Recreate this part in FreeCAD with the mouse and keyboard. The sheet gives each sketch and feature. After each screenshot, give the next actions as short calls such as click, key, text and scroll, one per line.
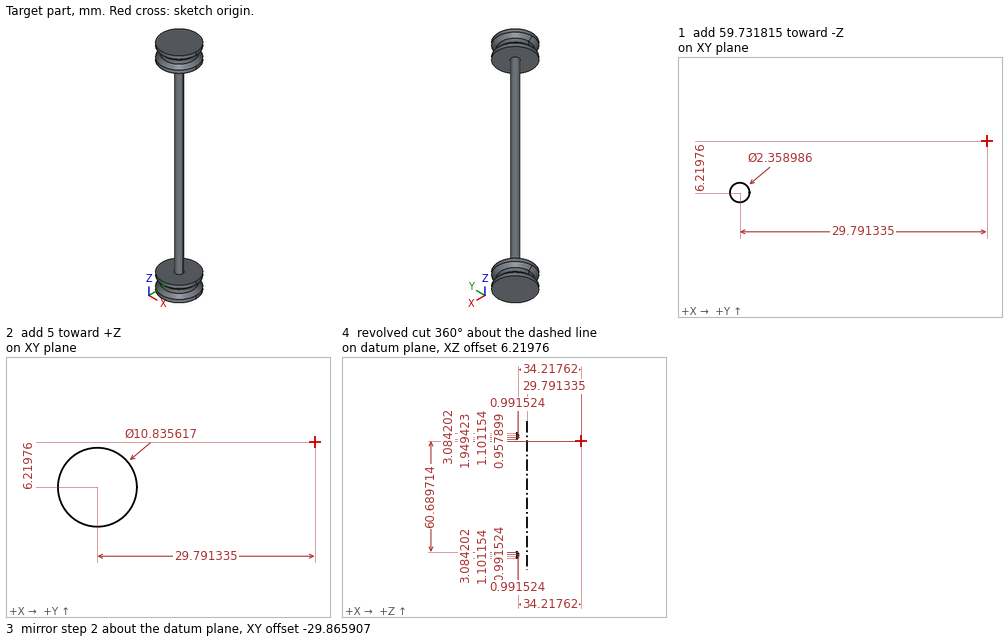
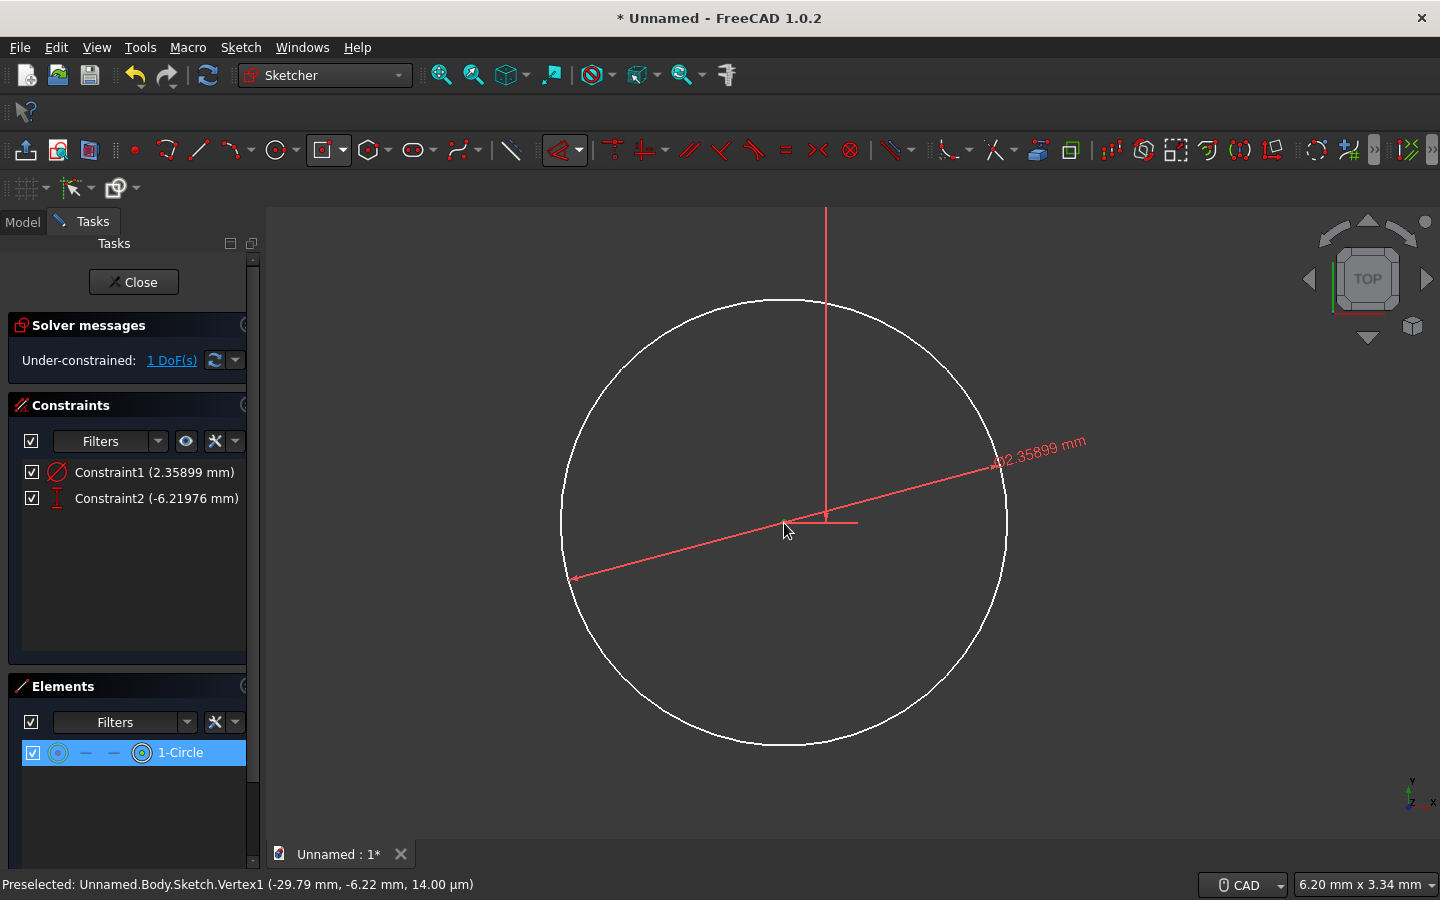
click(582, 150)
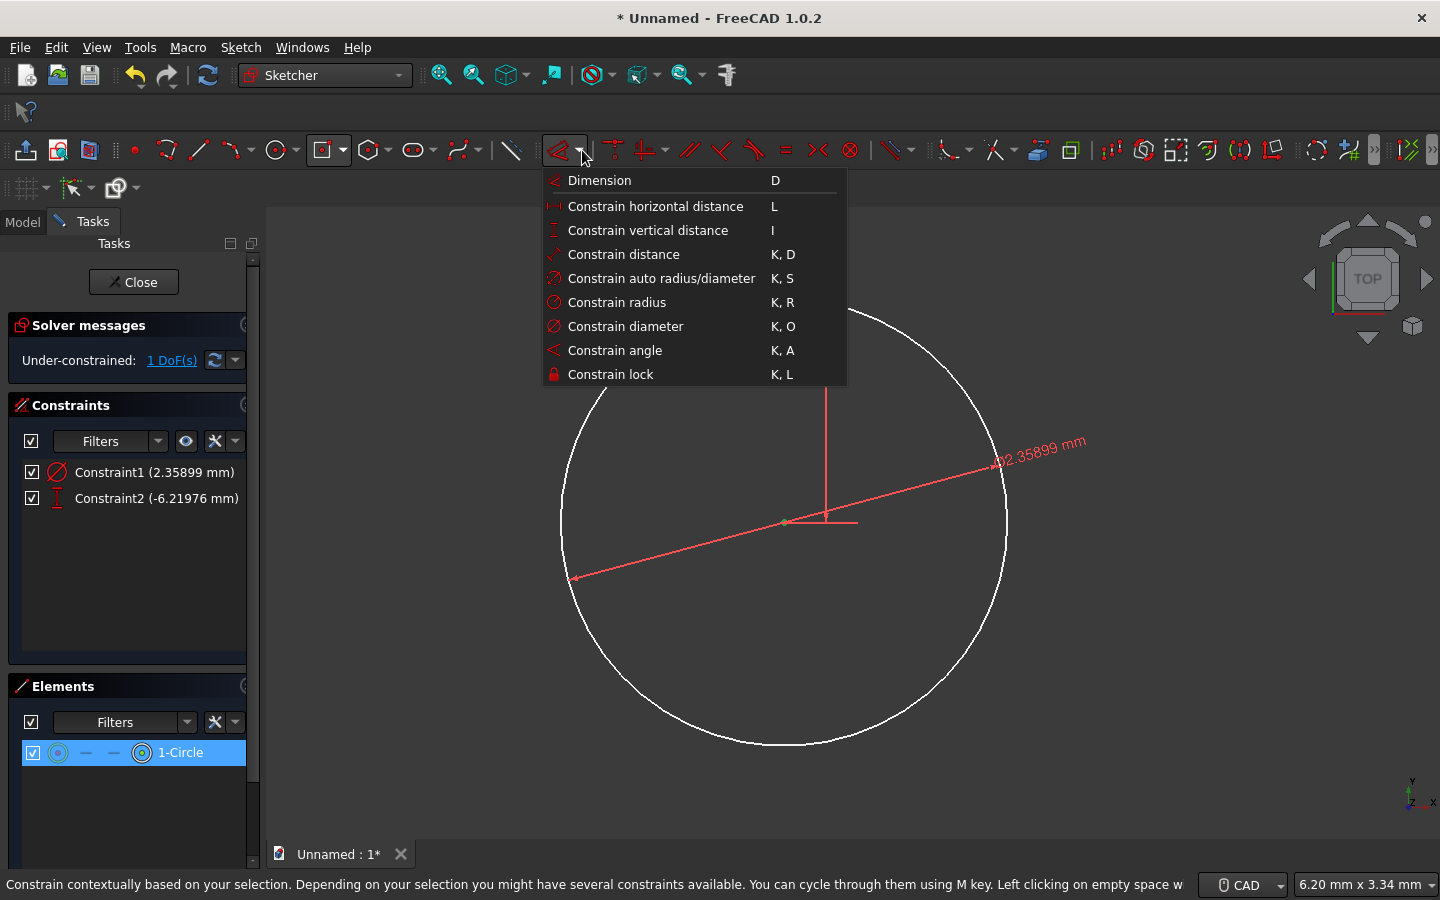
click(695, 206)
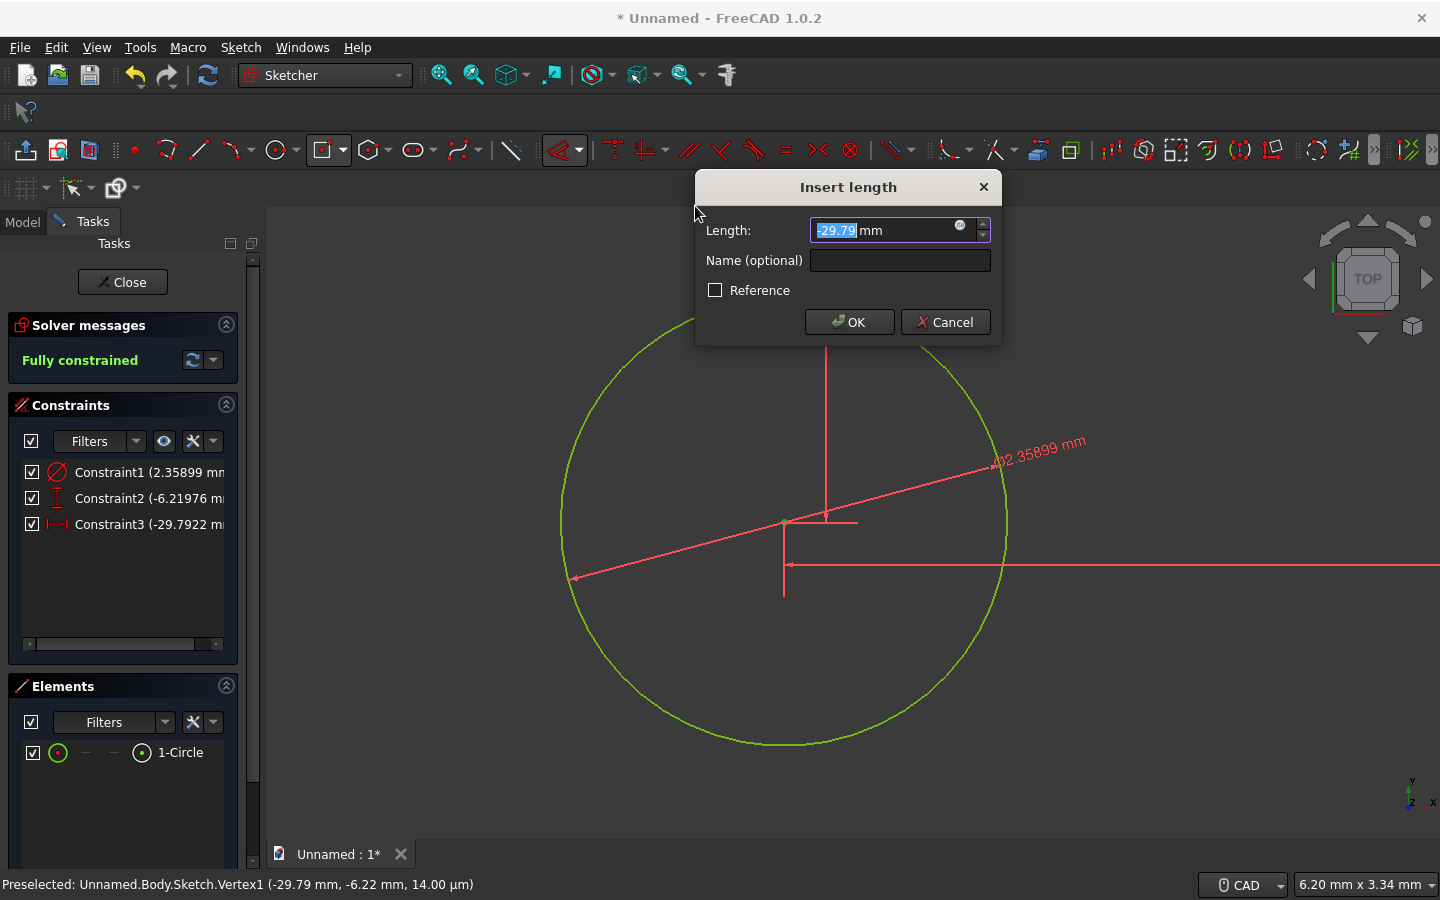
text(-29.791335)
key(Return)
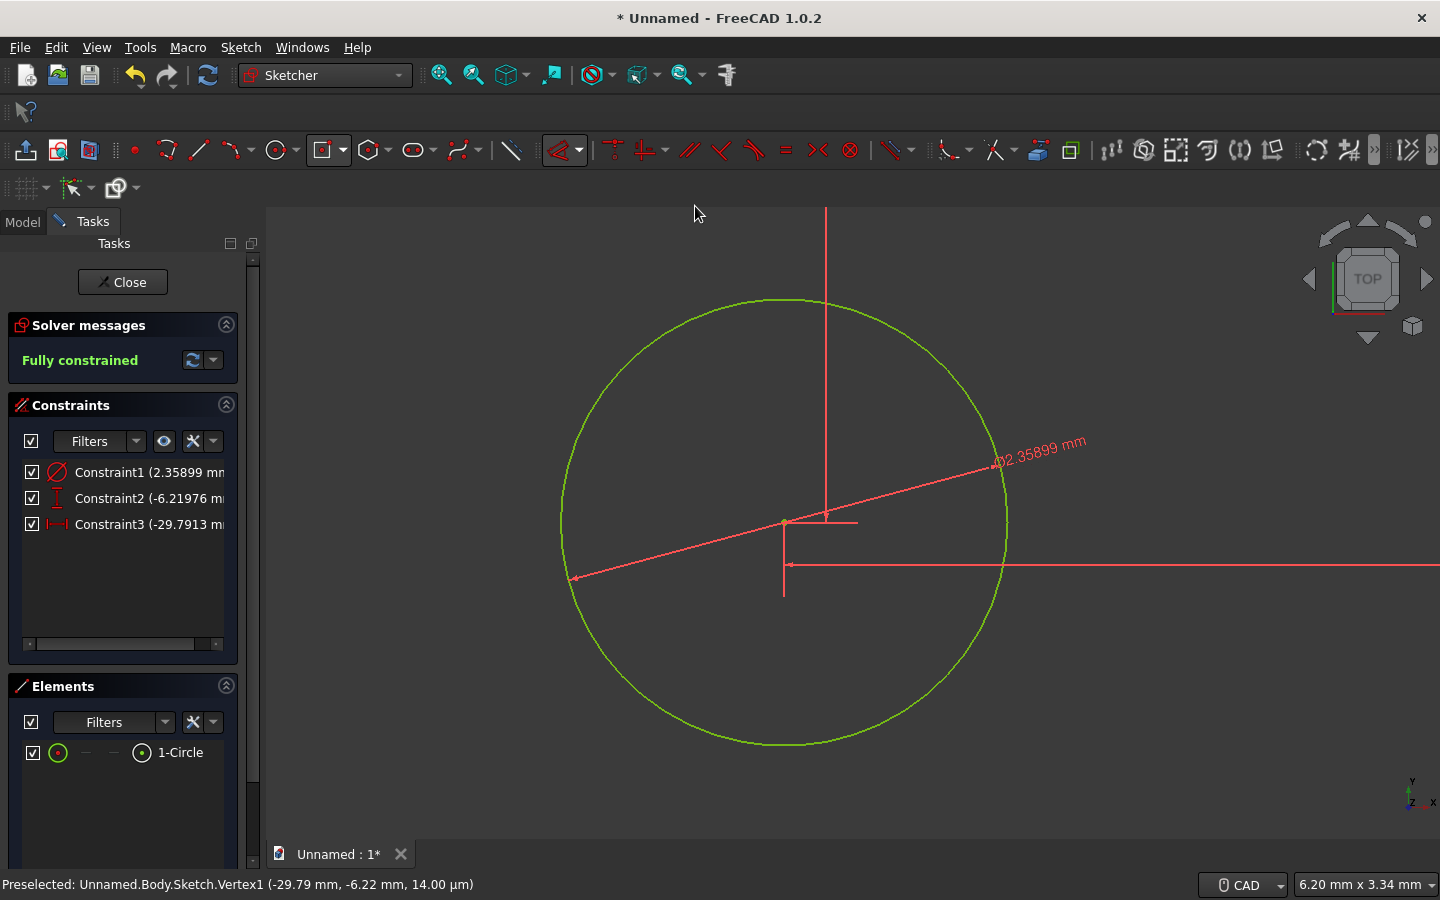
click(123, 282)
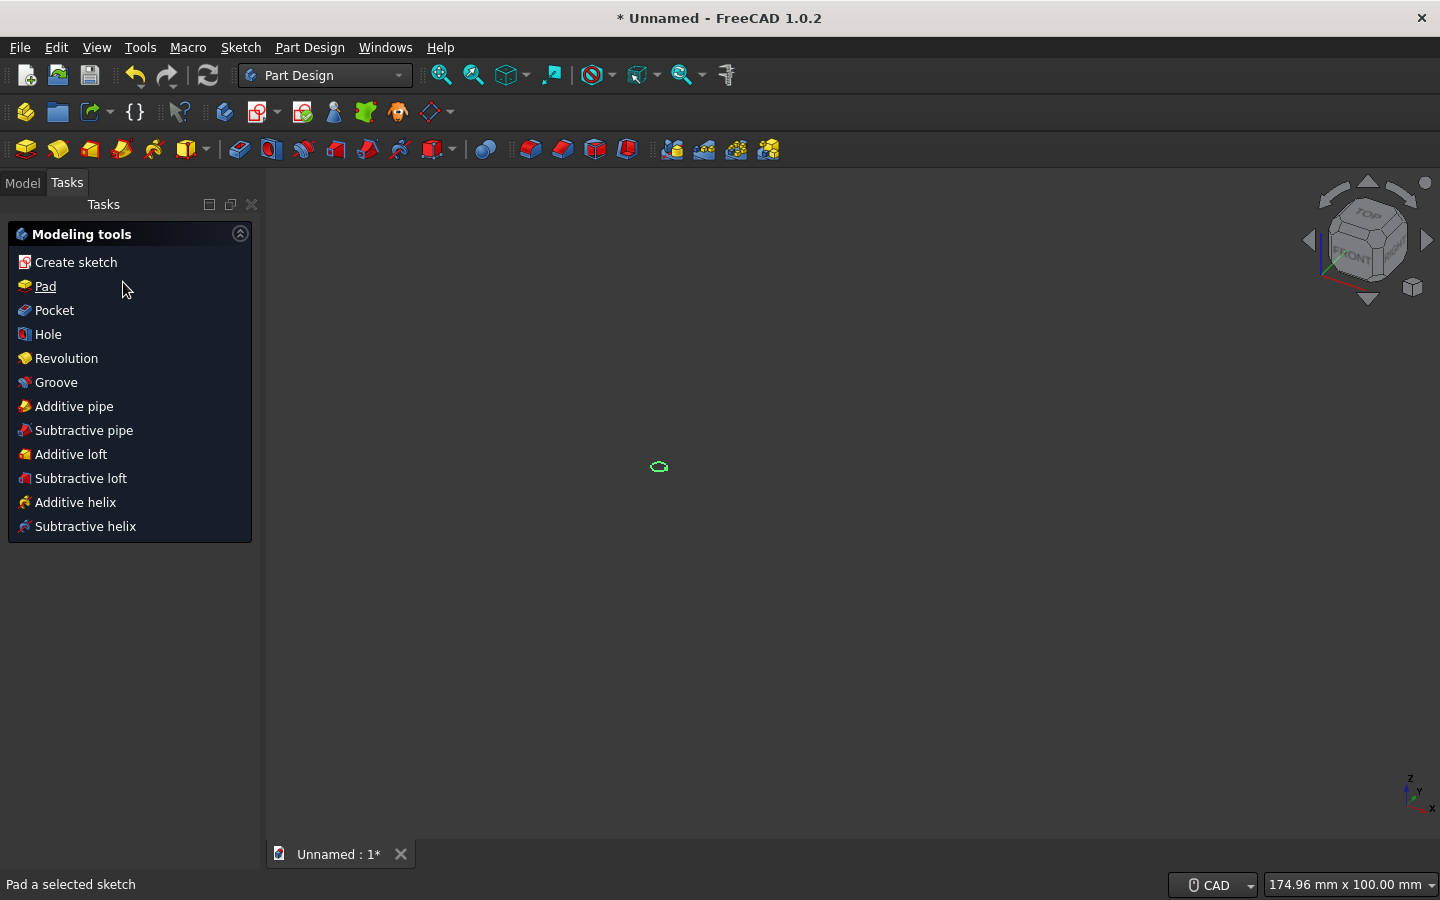
click(26, 150)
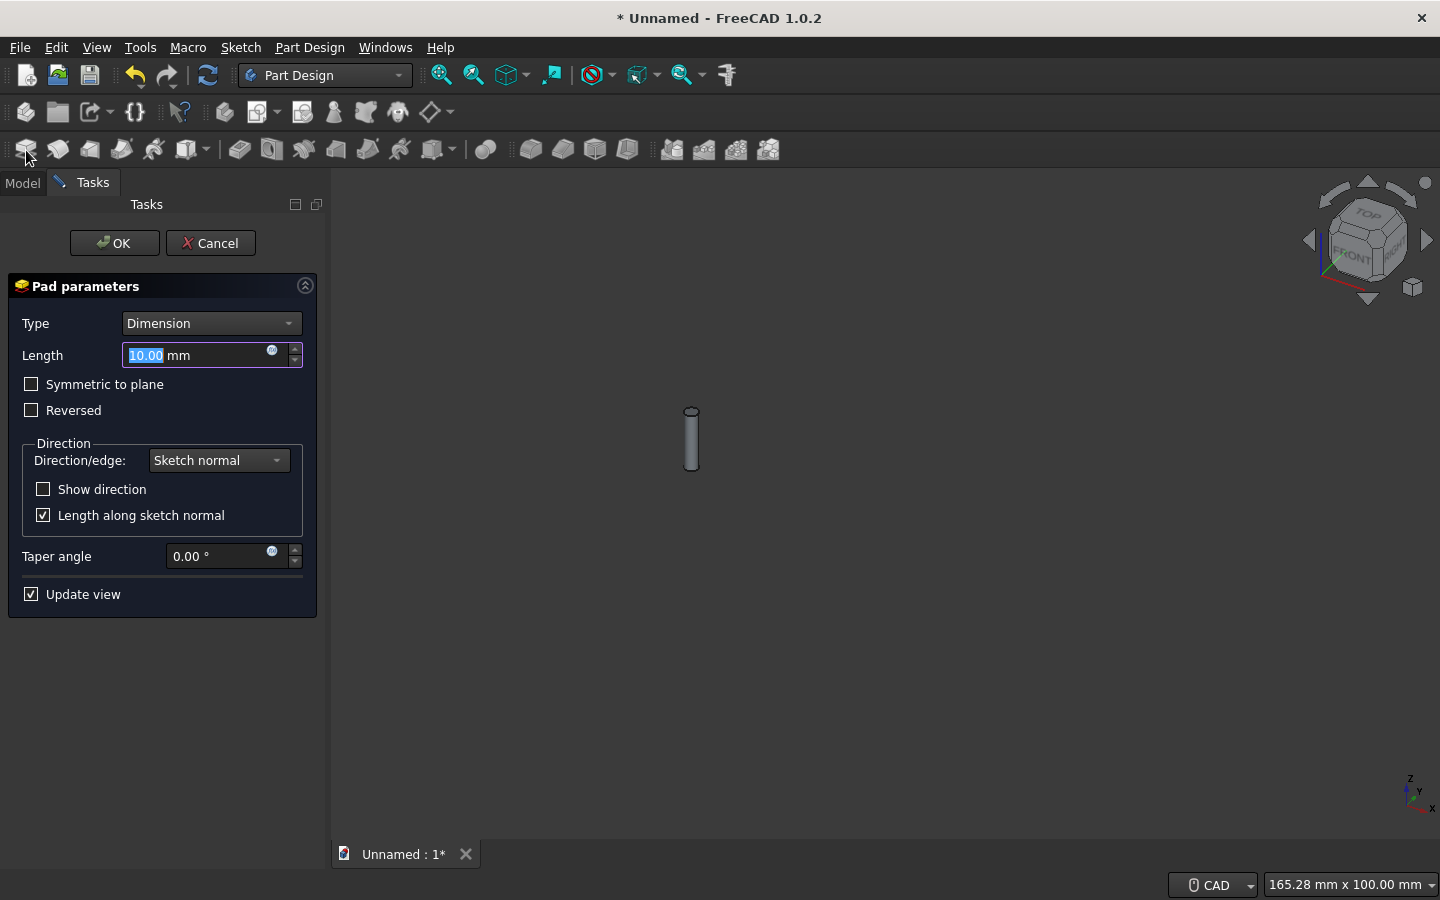
text(59.731815)
key(Tab)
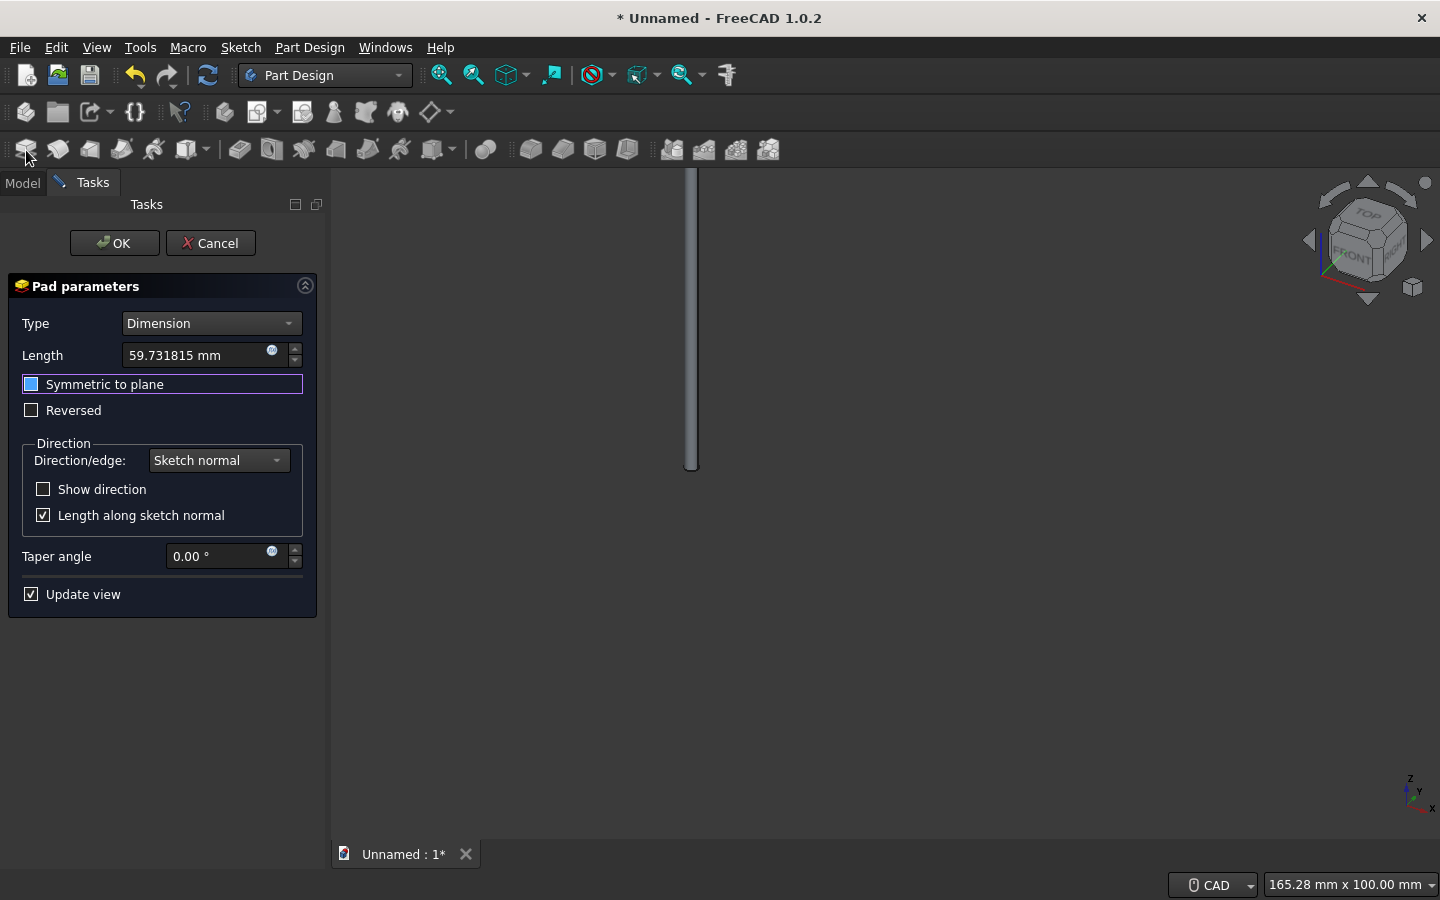
click(30, 410)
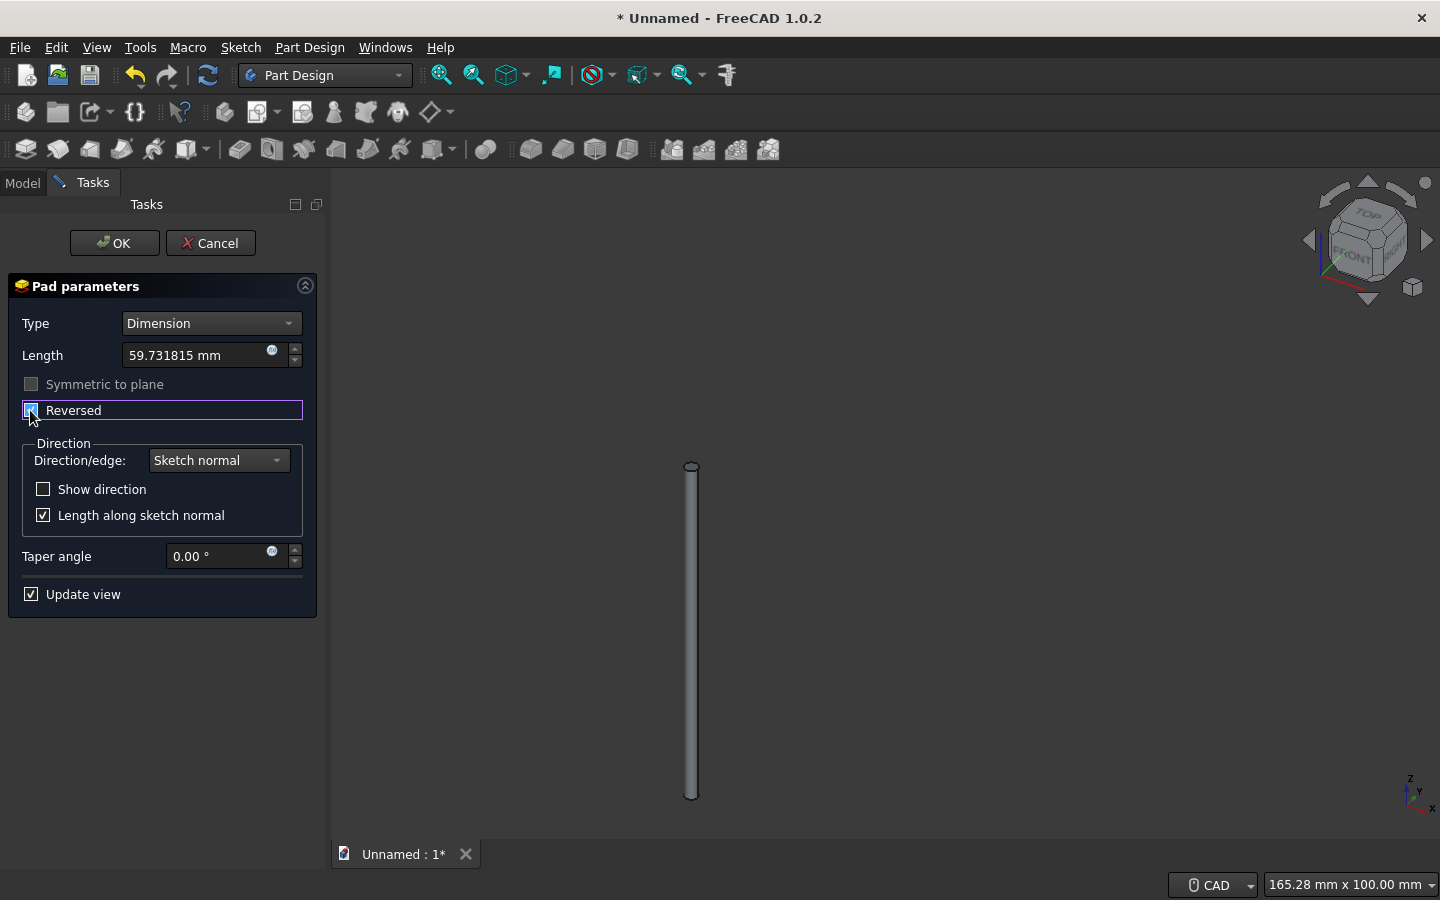
click(115, 243)